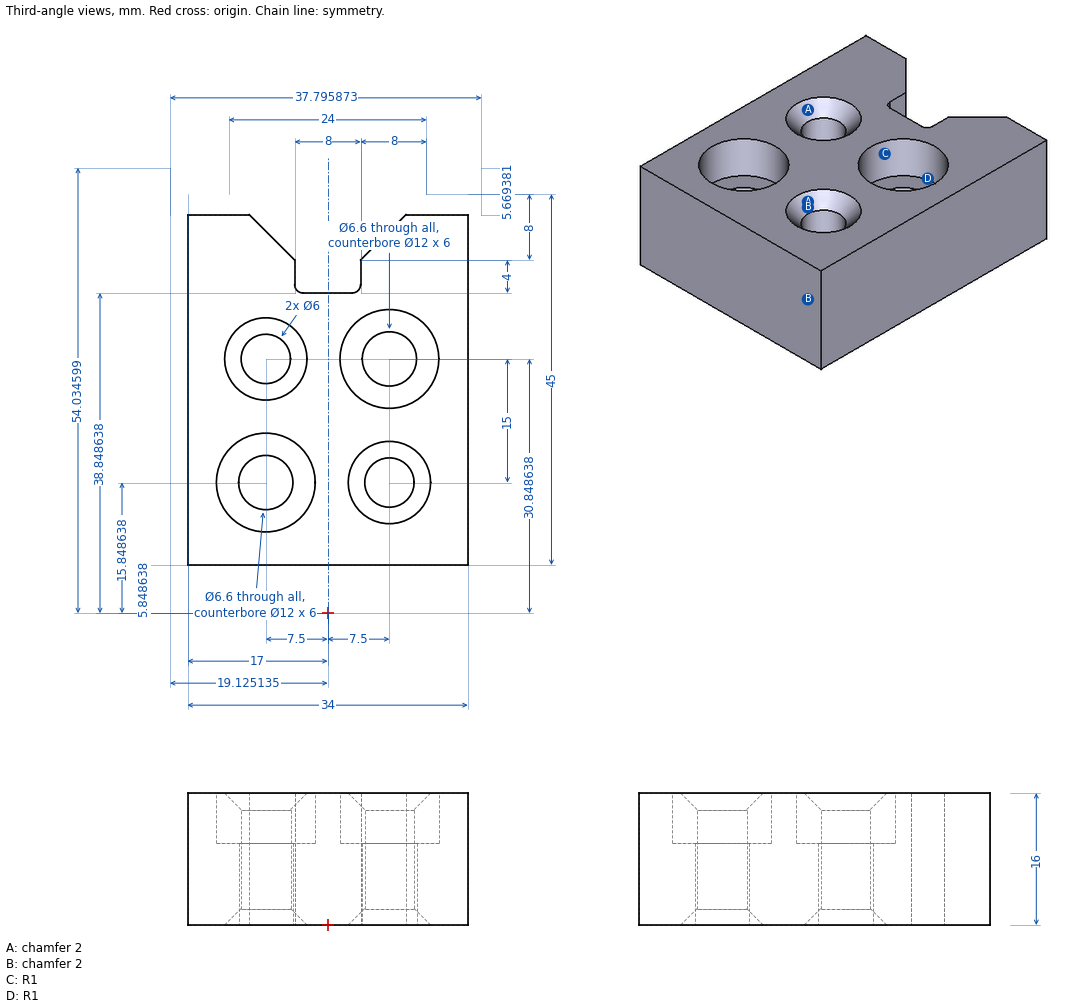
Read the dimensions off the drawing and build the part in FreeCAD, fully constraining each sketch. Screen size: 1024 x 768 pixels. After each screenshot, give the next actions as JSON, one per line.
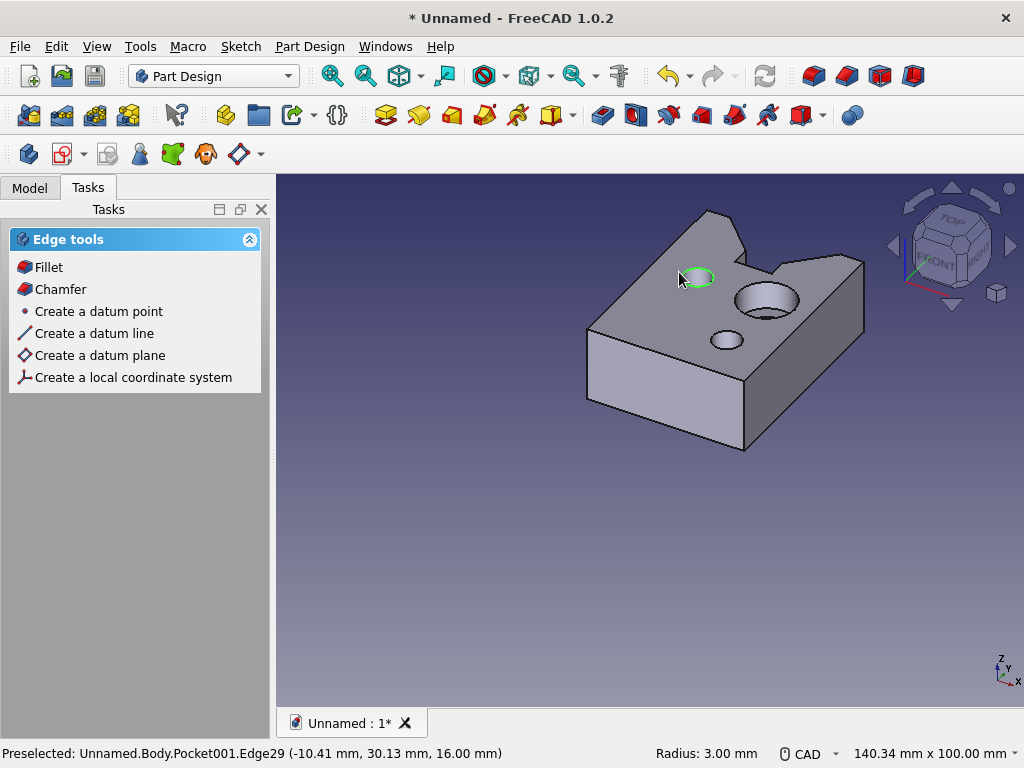
{"action": "left_click", "coordinate": [713, 335], "text": "ctrl"}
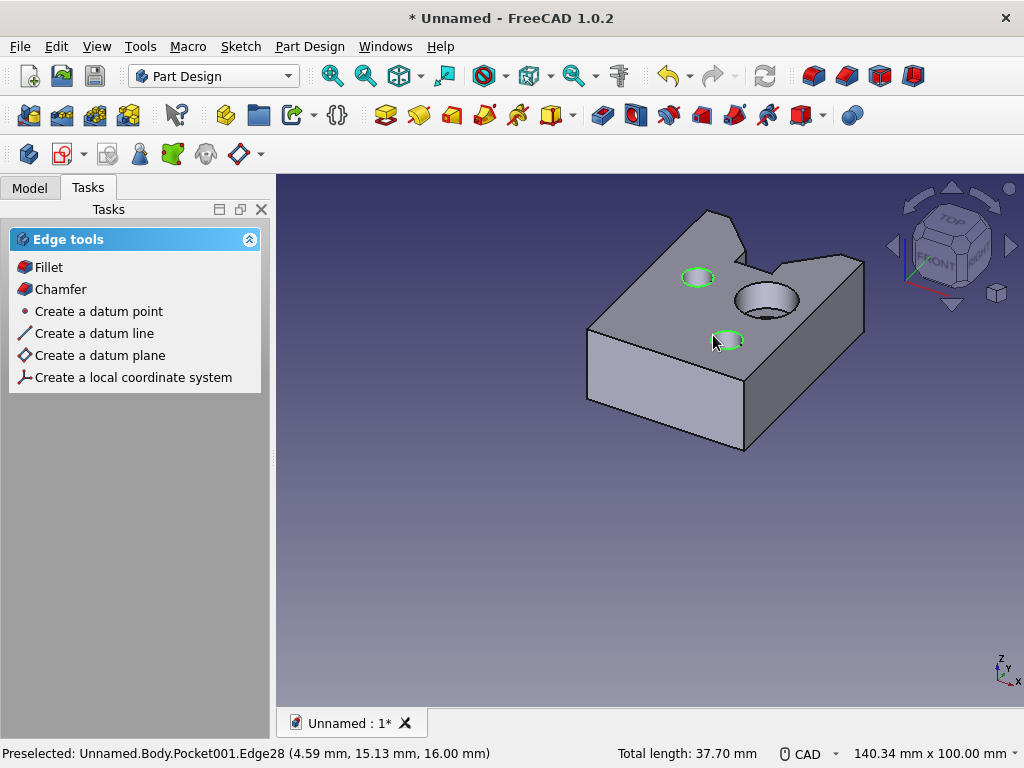
{"action": "left_click", "coordinate": [847, 76]}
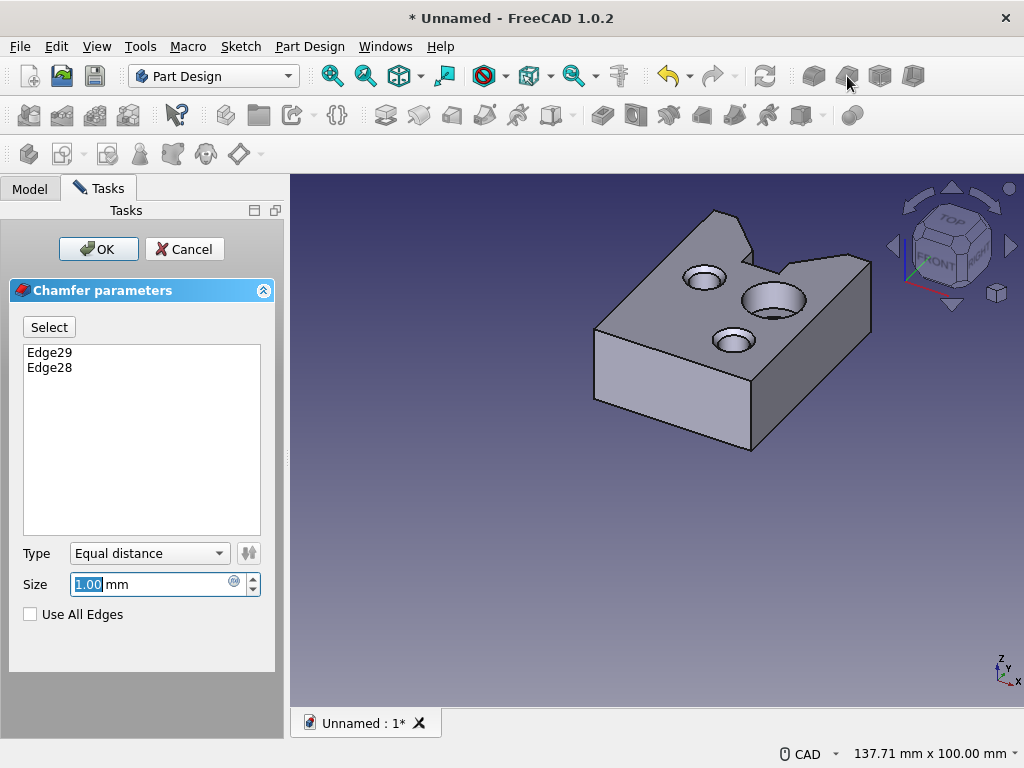
{"action": "type", "text": "2"}
{"action": "key", "text": "Tab"}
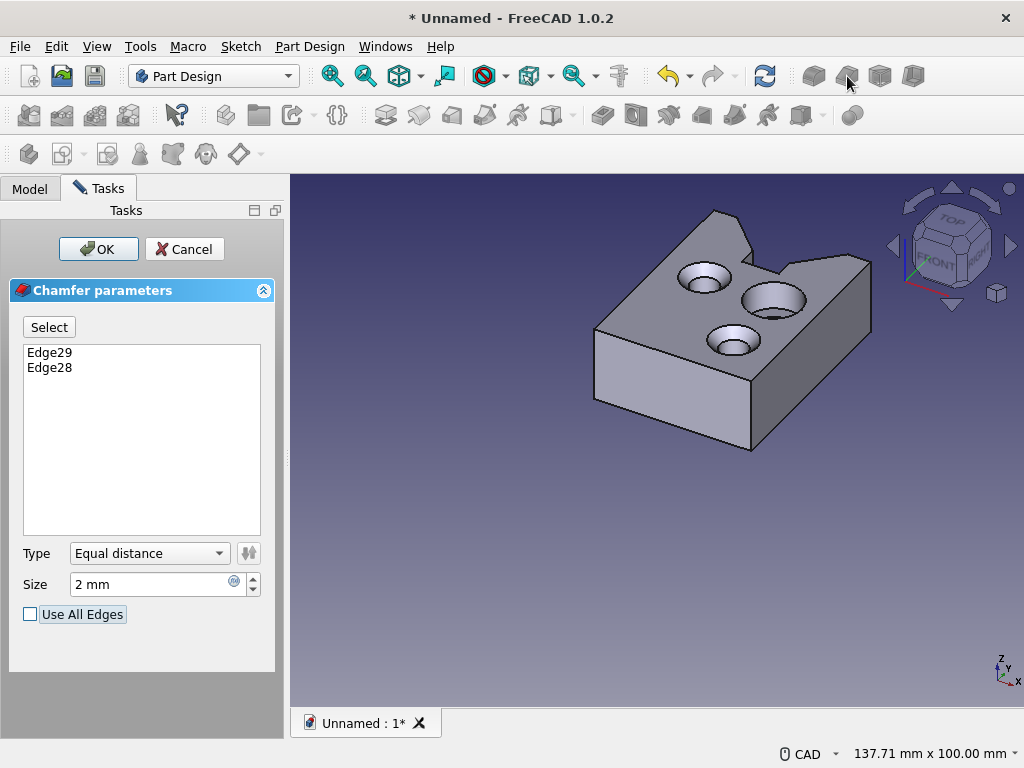
{"action": "left_click", "coordinate": [99, 249]}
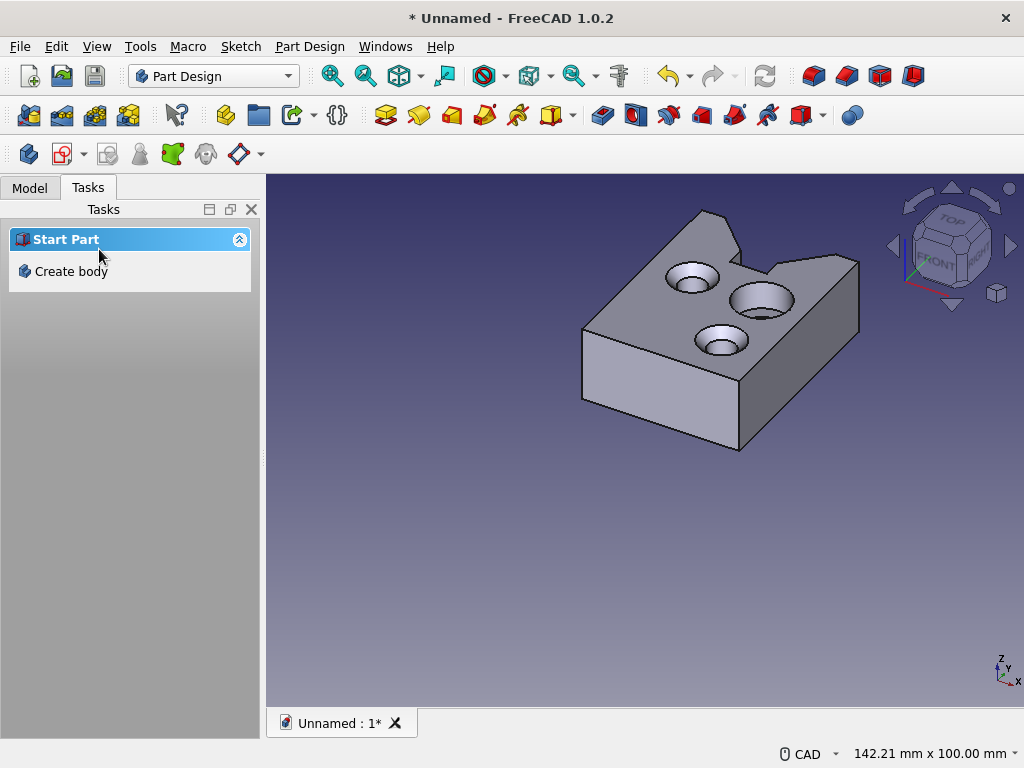
{"action": "key", "text": "0"}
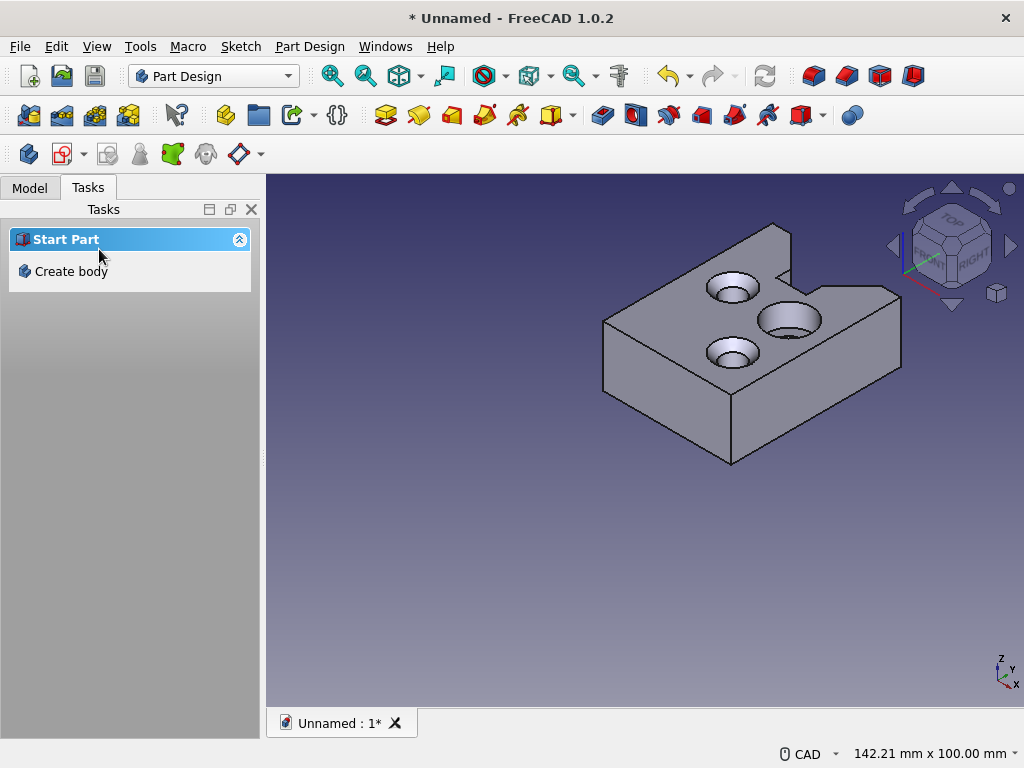
{"action": "key", "text": "2"}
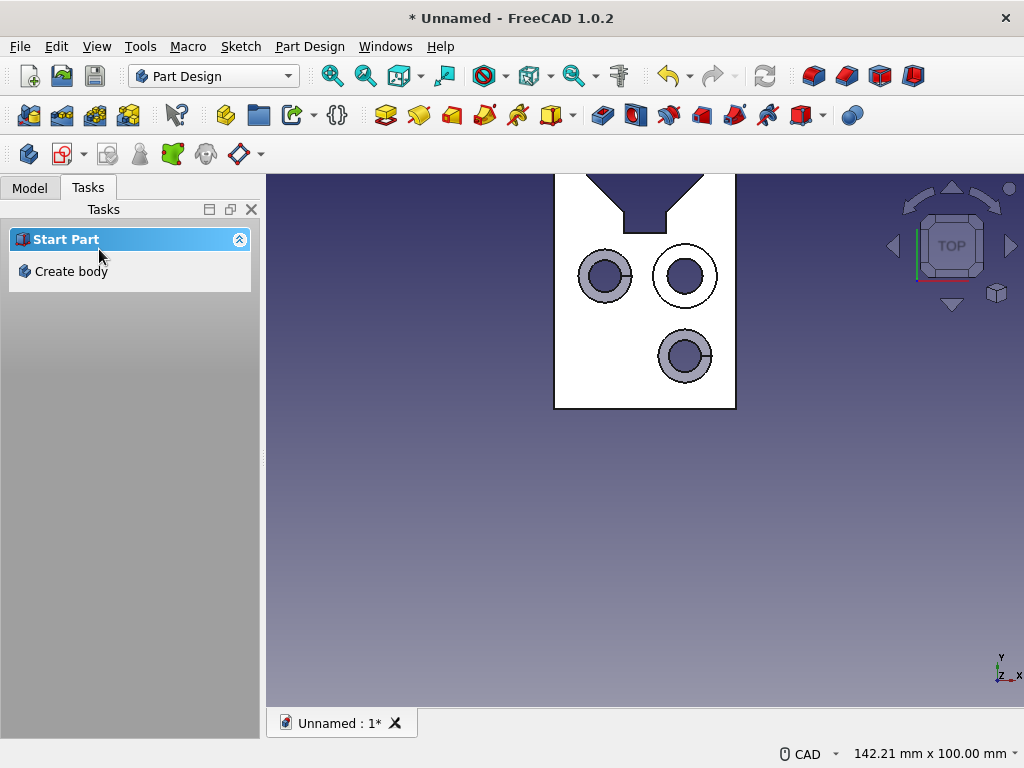
{"action": "left_click", "coordinate": [333, 76]}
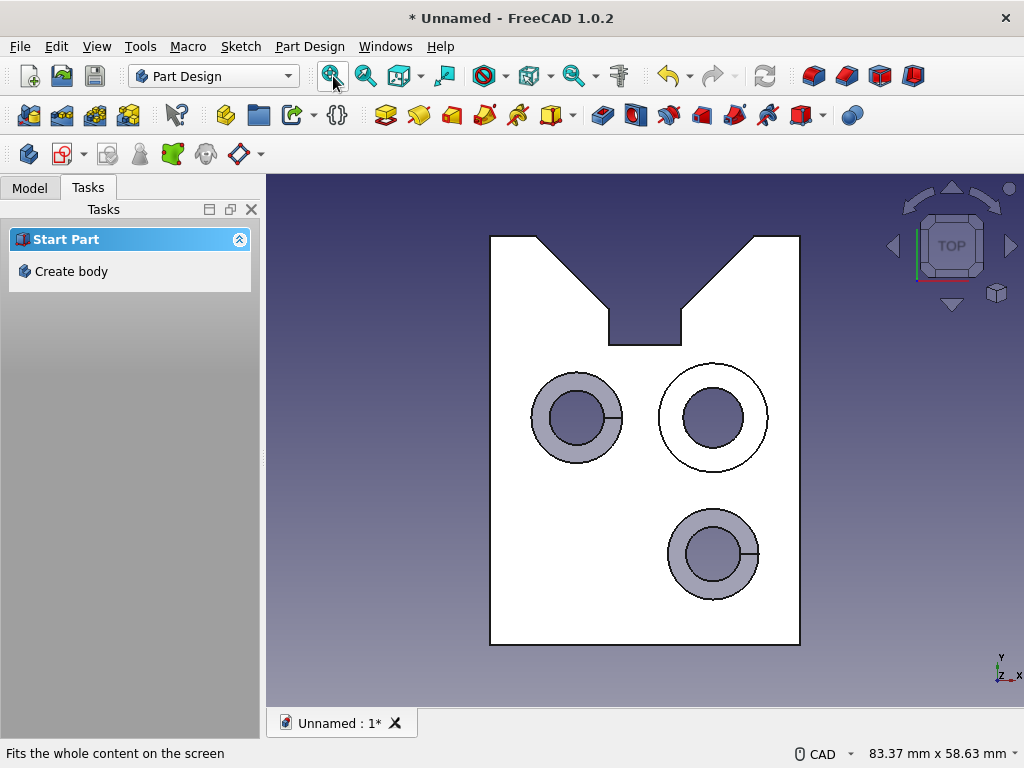
{"action": "key", "text": "1"}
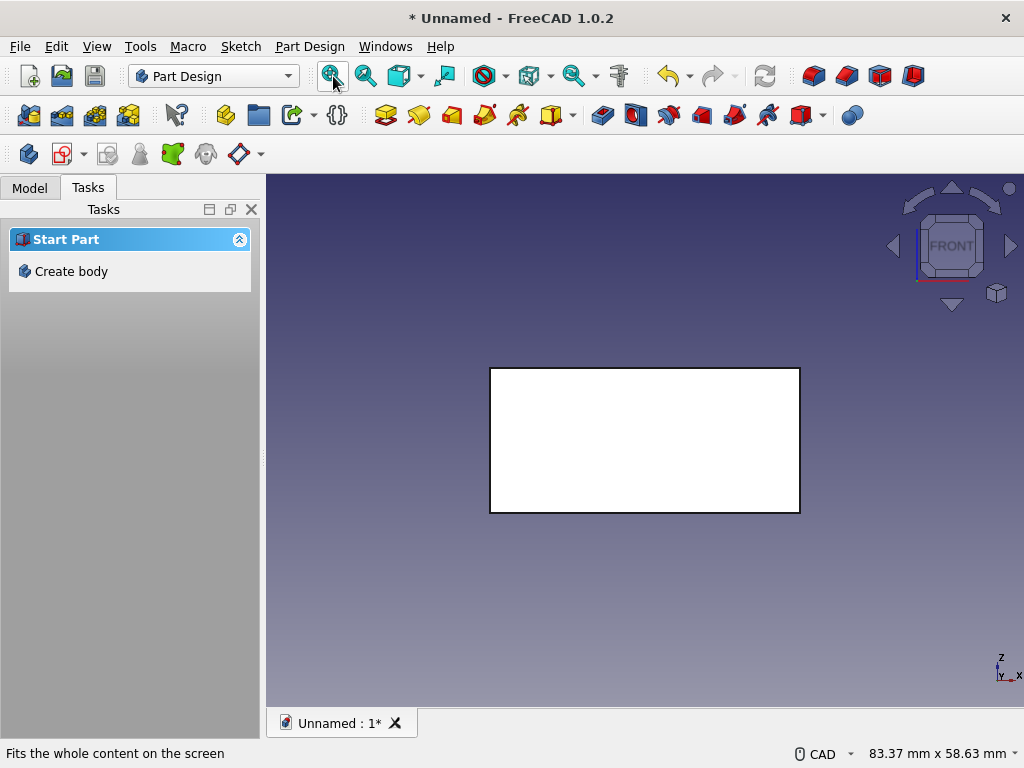
{"action": "left_click", "coordinate": [333, 76]}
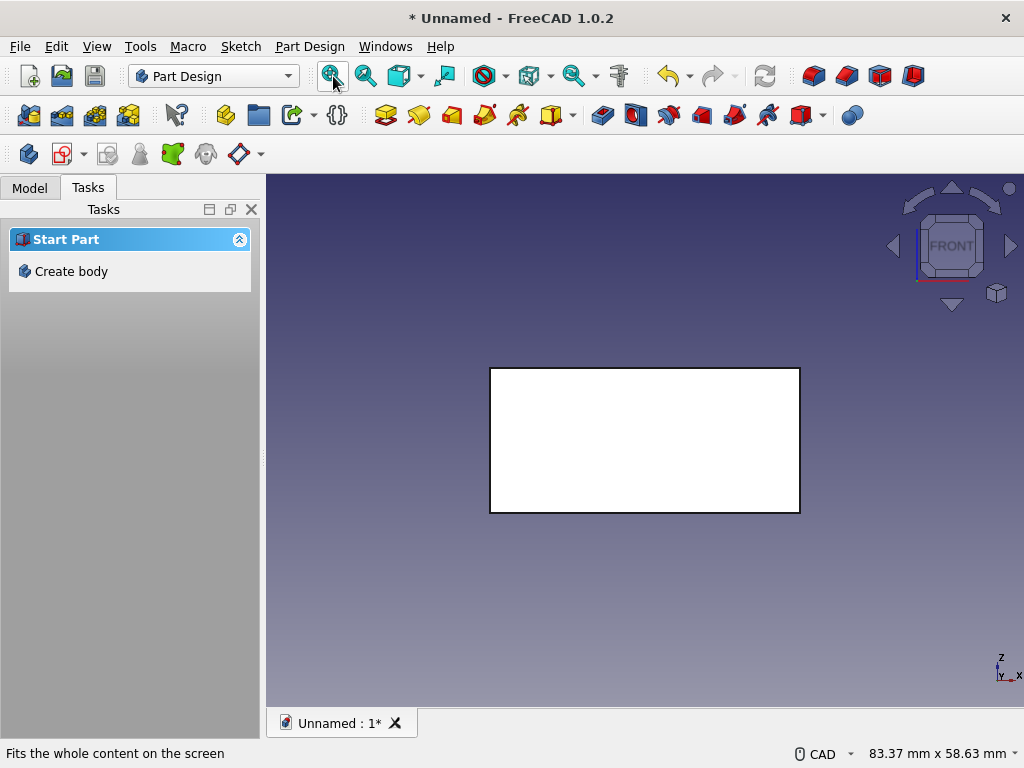
{"action": "key", "text": "3"}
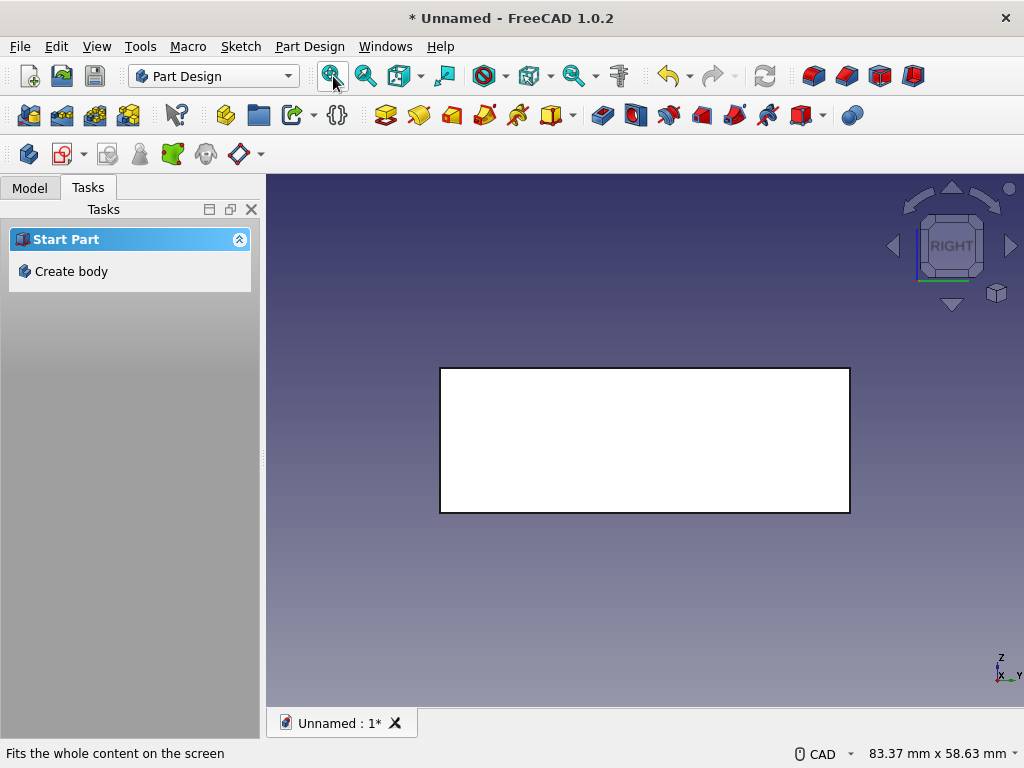
{"action": "key", "text": "5"}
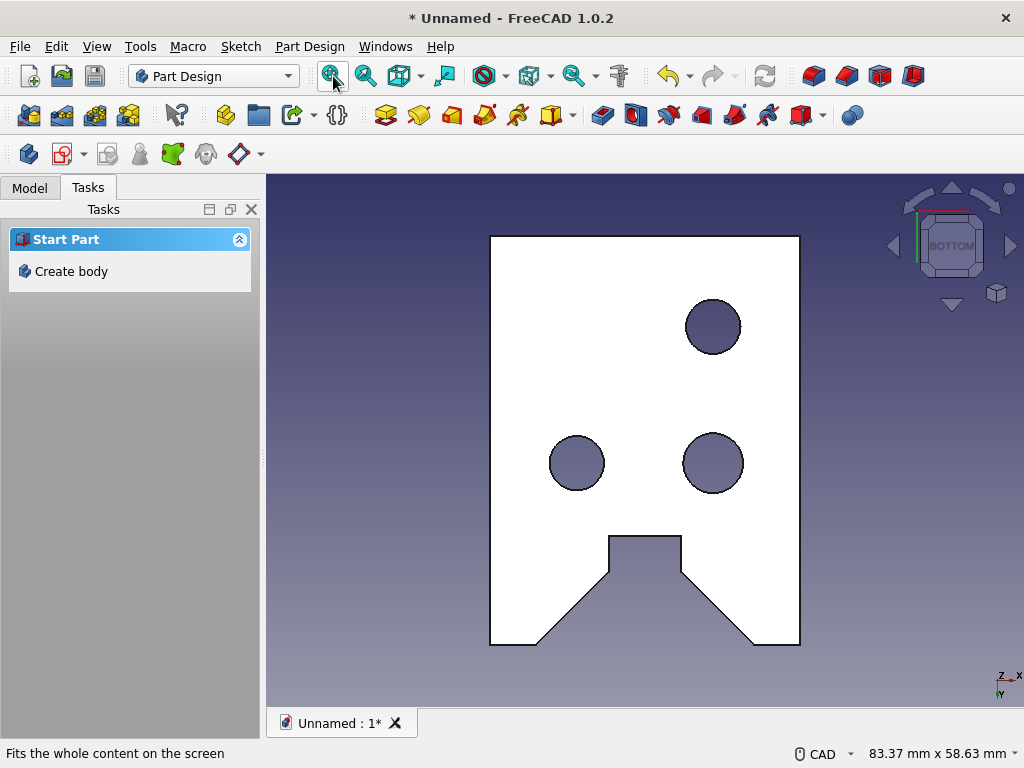
{"action": "left_click", "coordinate": [550, 462]}